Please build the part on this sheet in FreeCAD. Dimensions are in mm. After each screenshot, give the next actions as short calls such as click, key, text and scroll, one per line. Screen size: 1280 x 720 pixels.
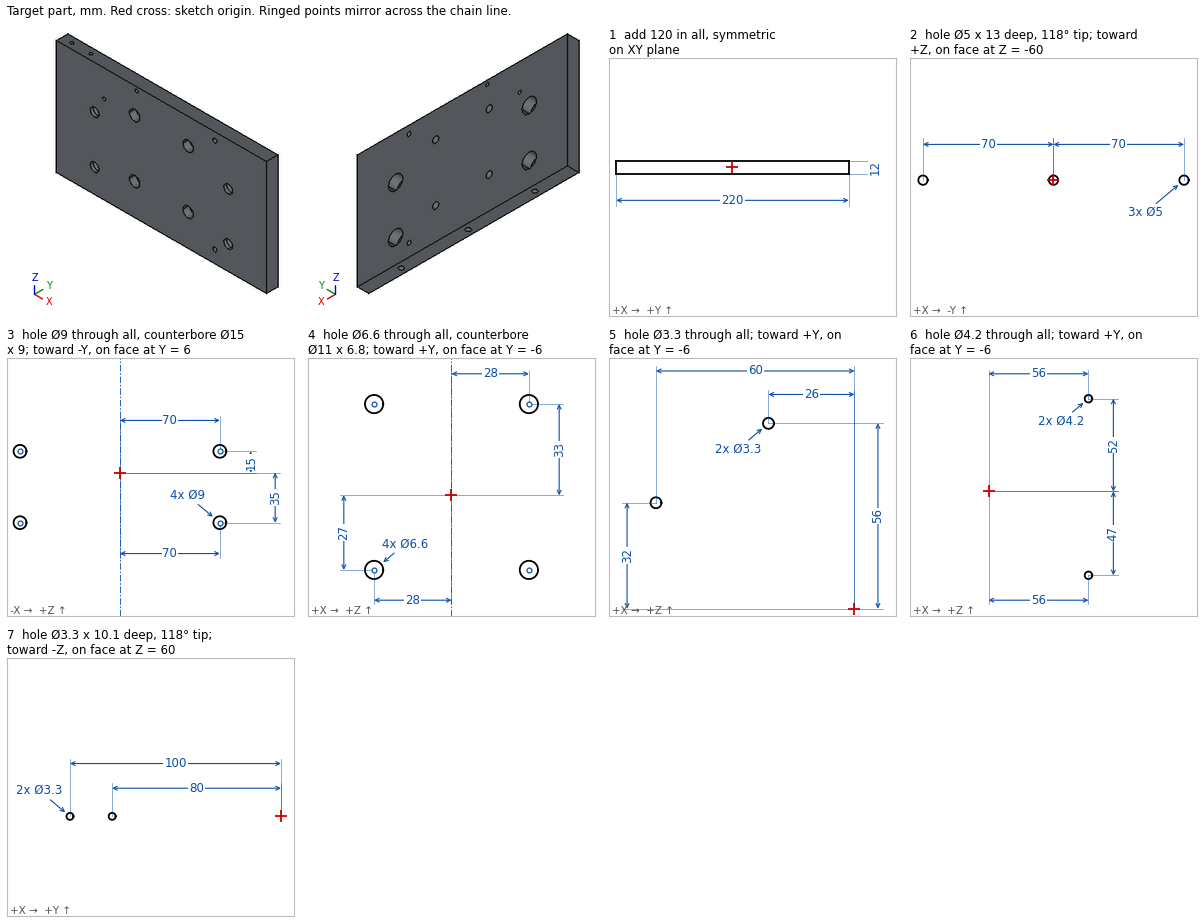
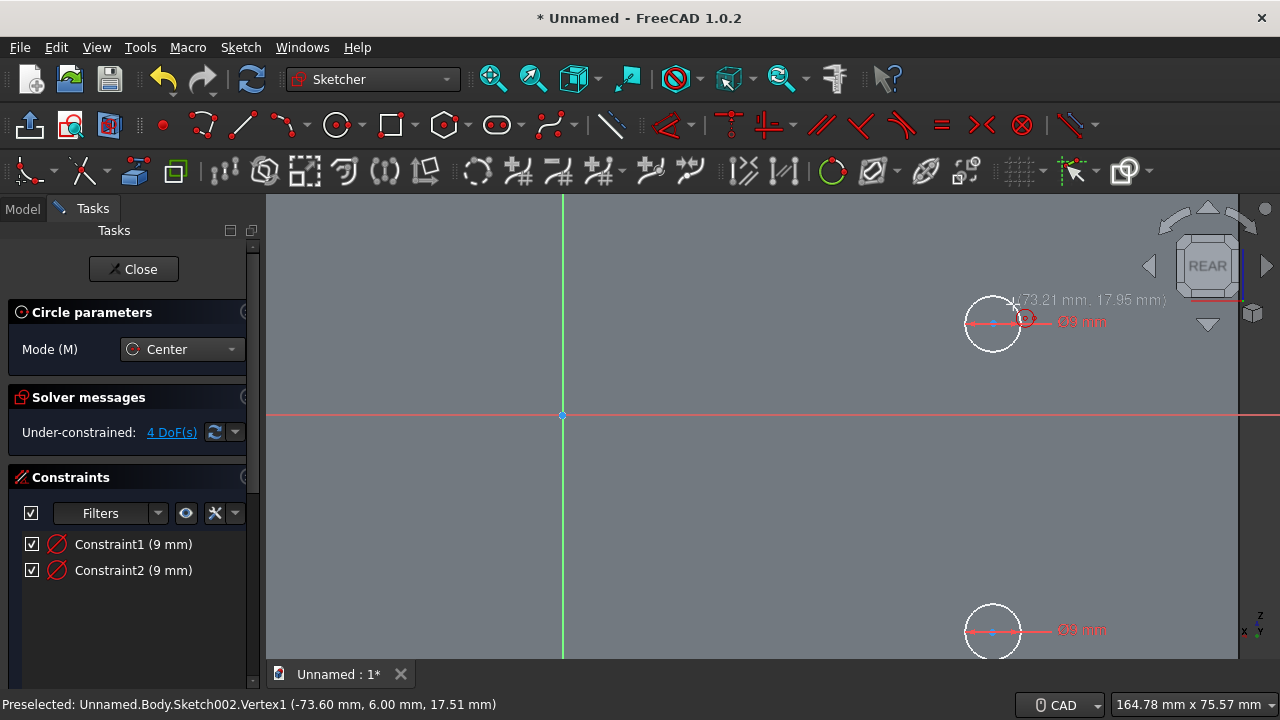
scroll(993, 324, down, 2)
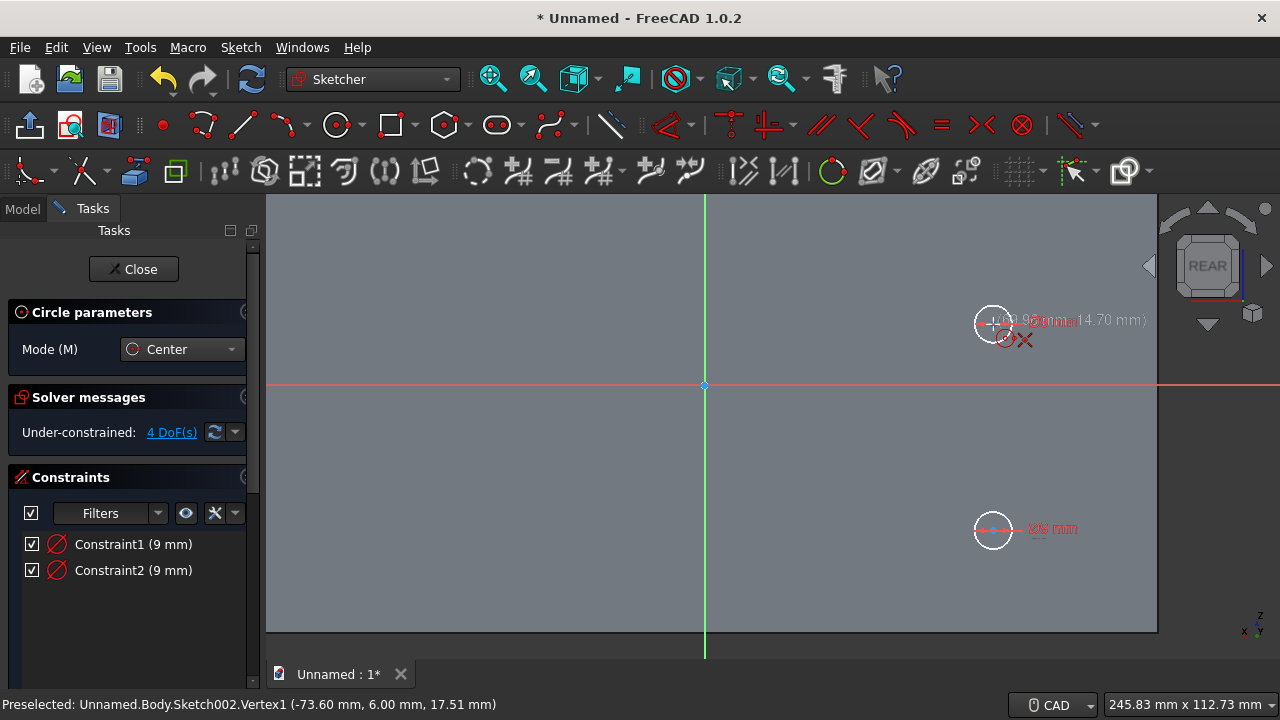
scroll(416, 530, up, 2)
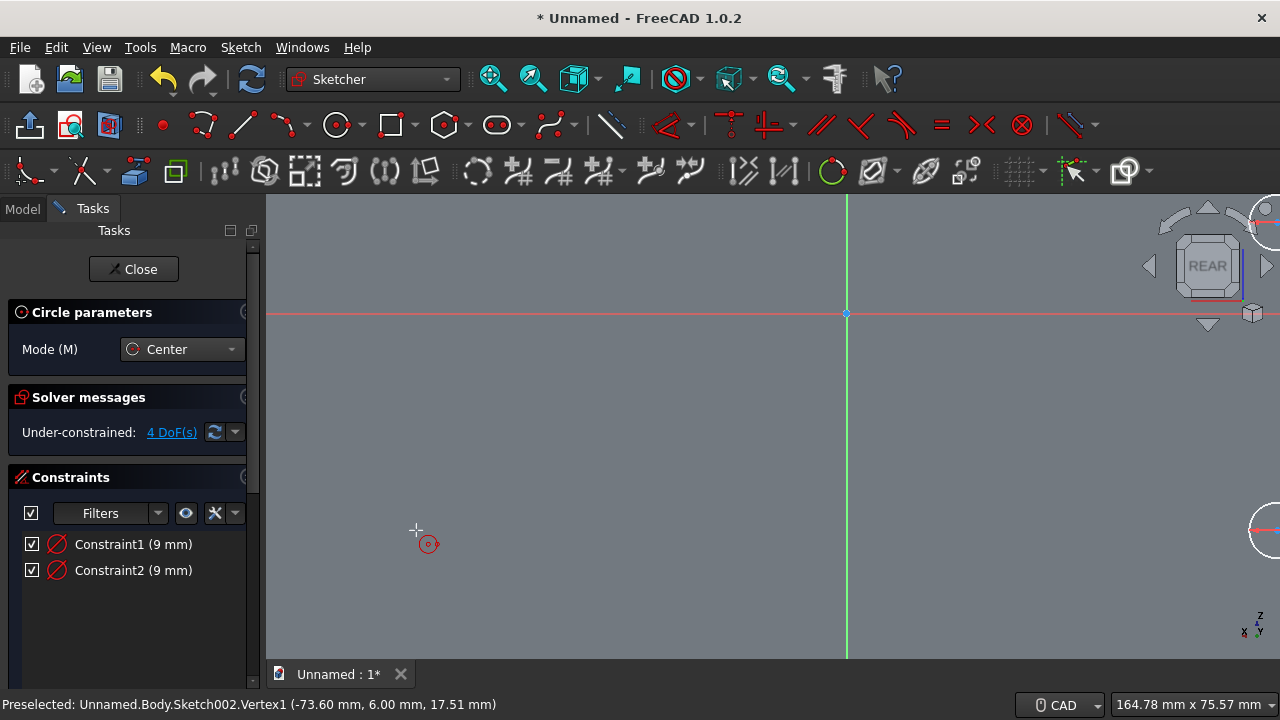
click(416, 529)
move(435, 510)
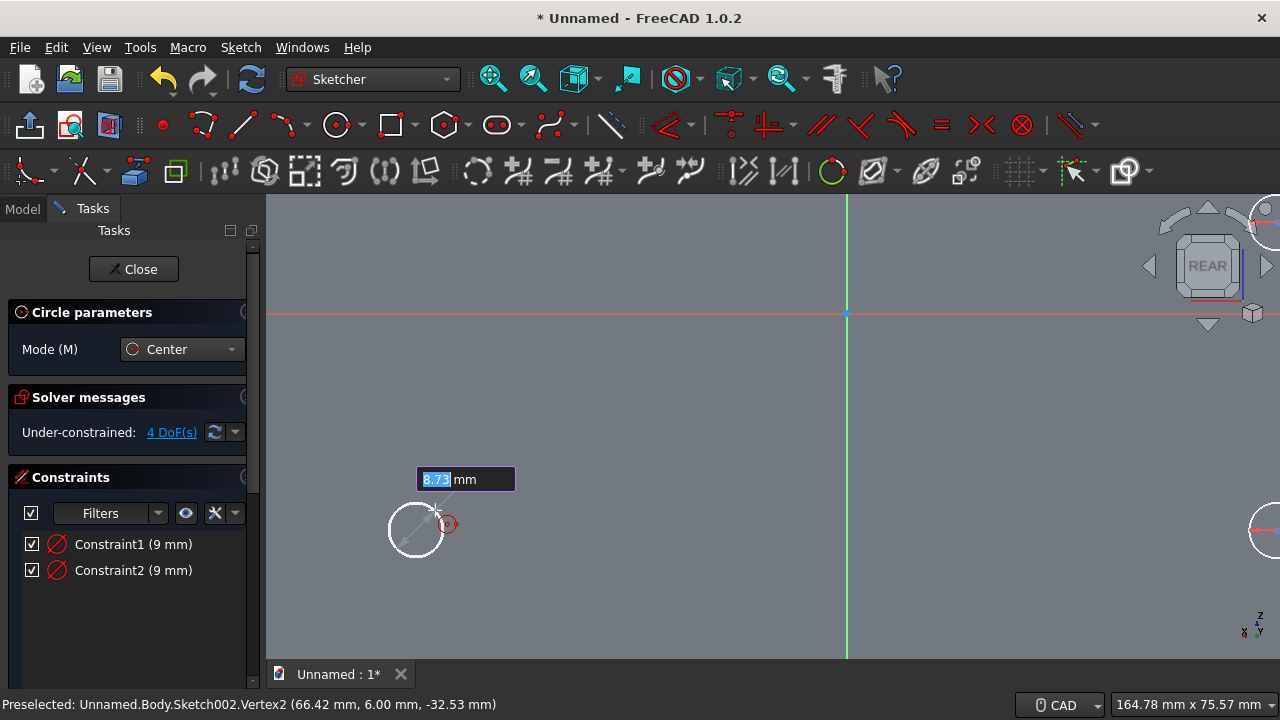
text(9)
key(Return)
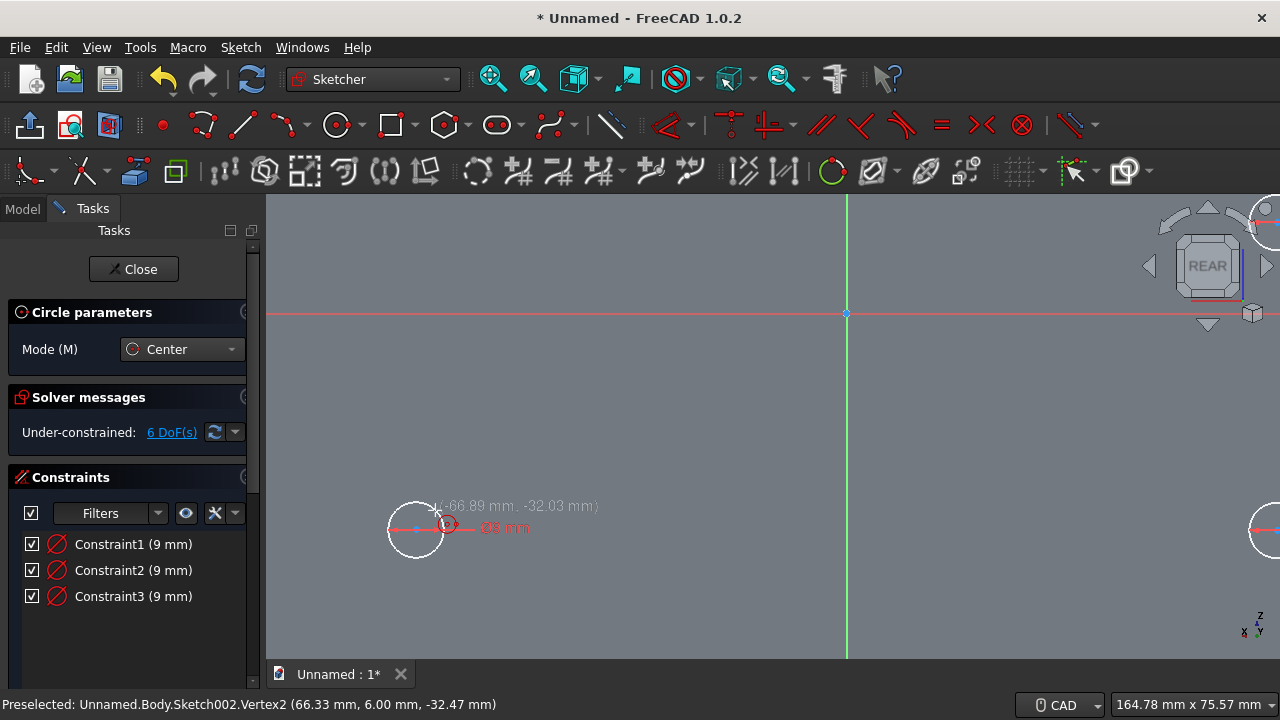
scroll(416, 530, down, 2)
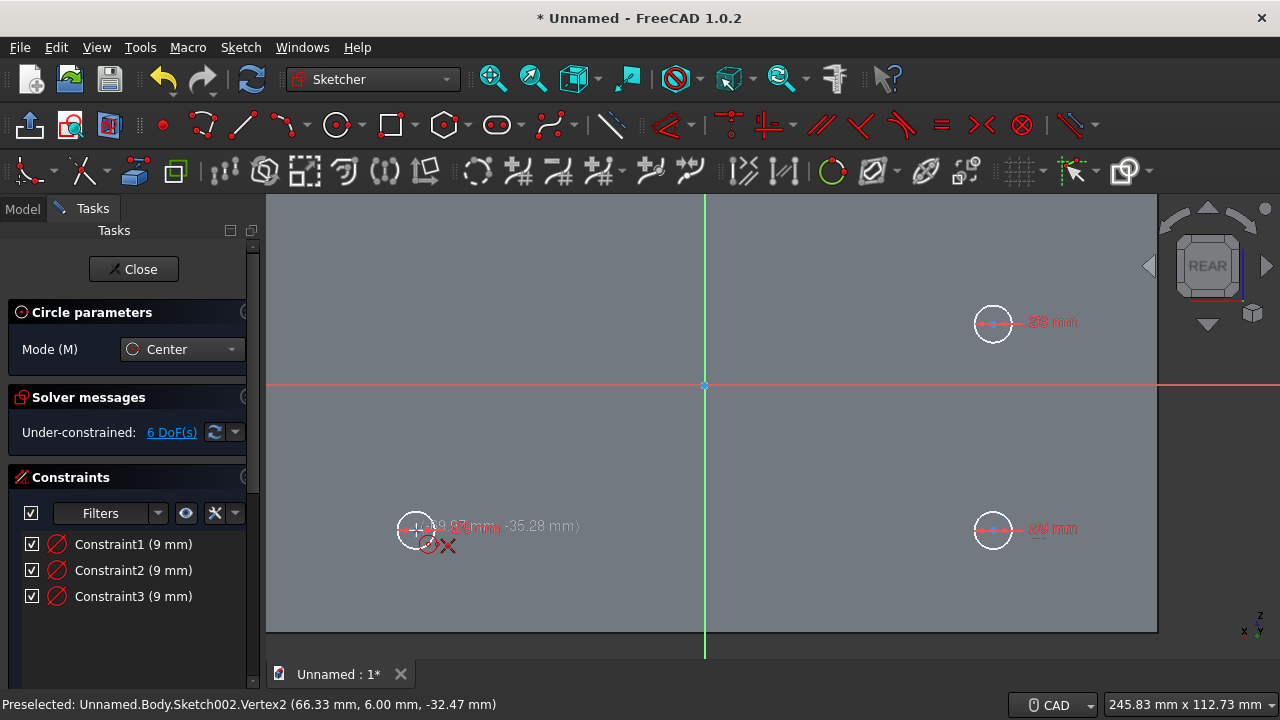
scroll(416, 324, up, 2)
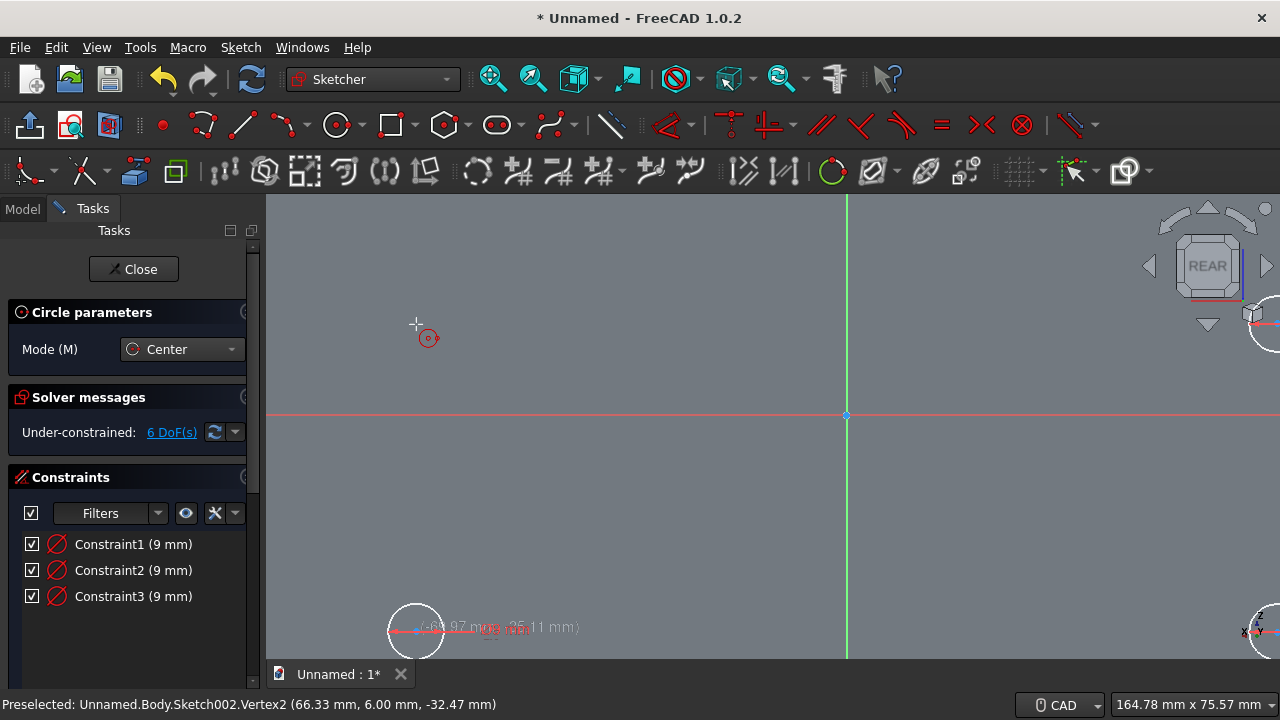
click(416, 323)
move(435, 304)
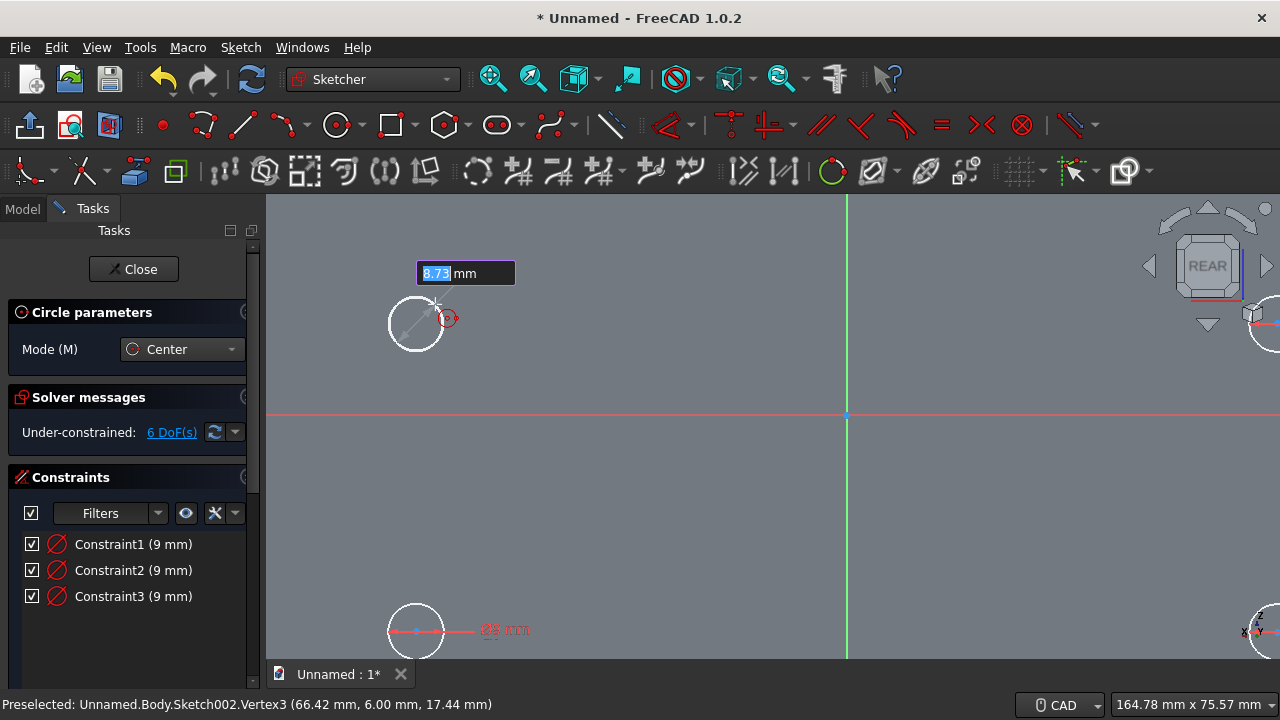
text(9)
key(Return)
key(Escape)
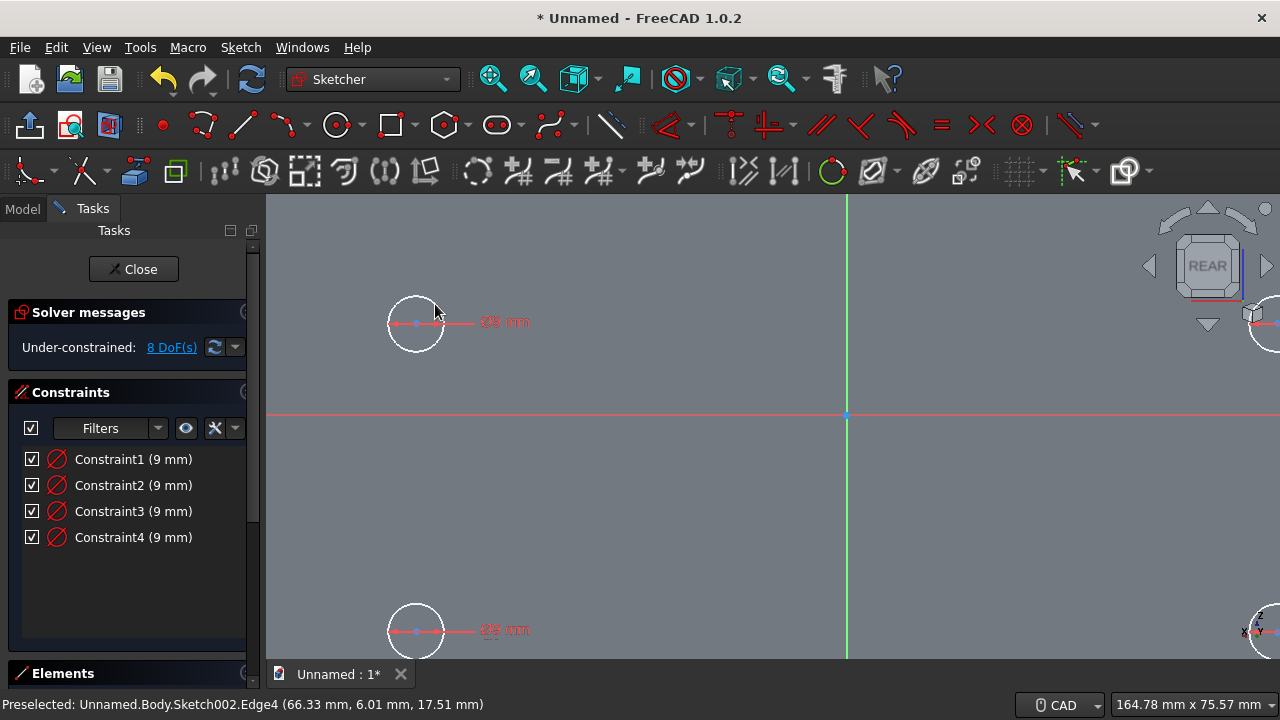
scroll(416, 324, down, 2)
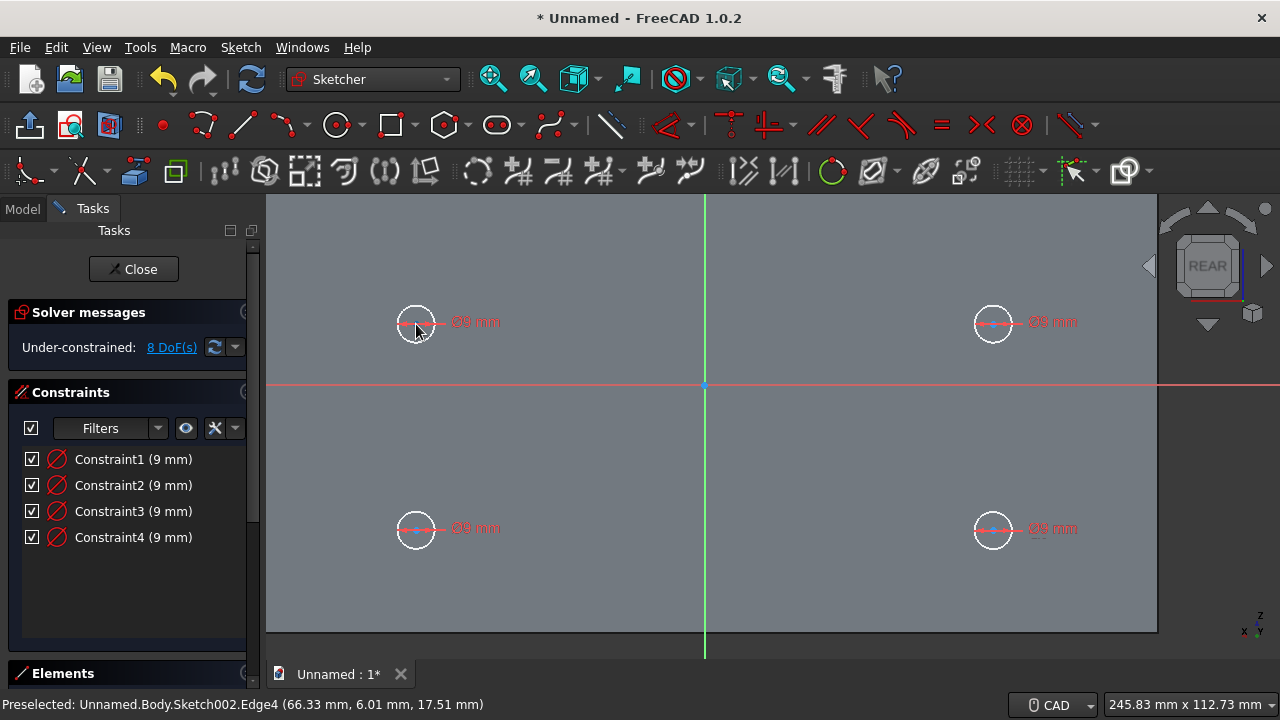
click(993, 531)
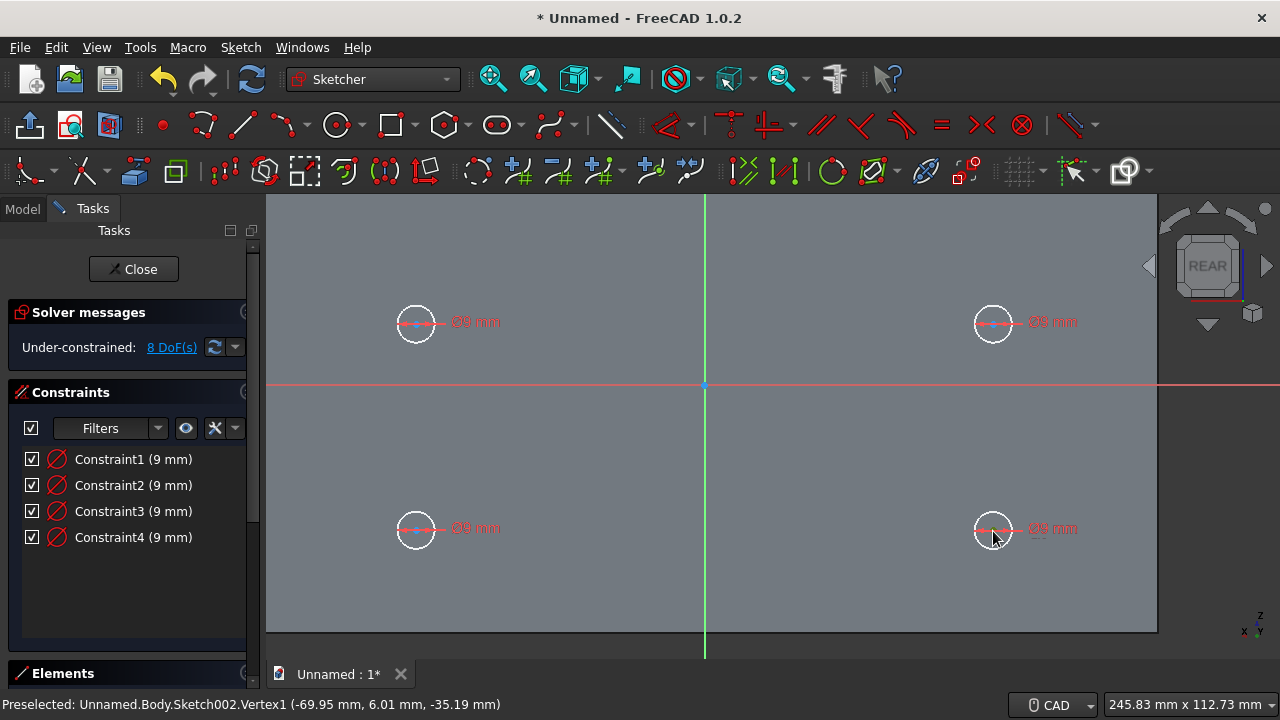
click(416, 530)